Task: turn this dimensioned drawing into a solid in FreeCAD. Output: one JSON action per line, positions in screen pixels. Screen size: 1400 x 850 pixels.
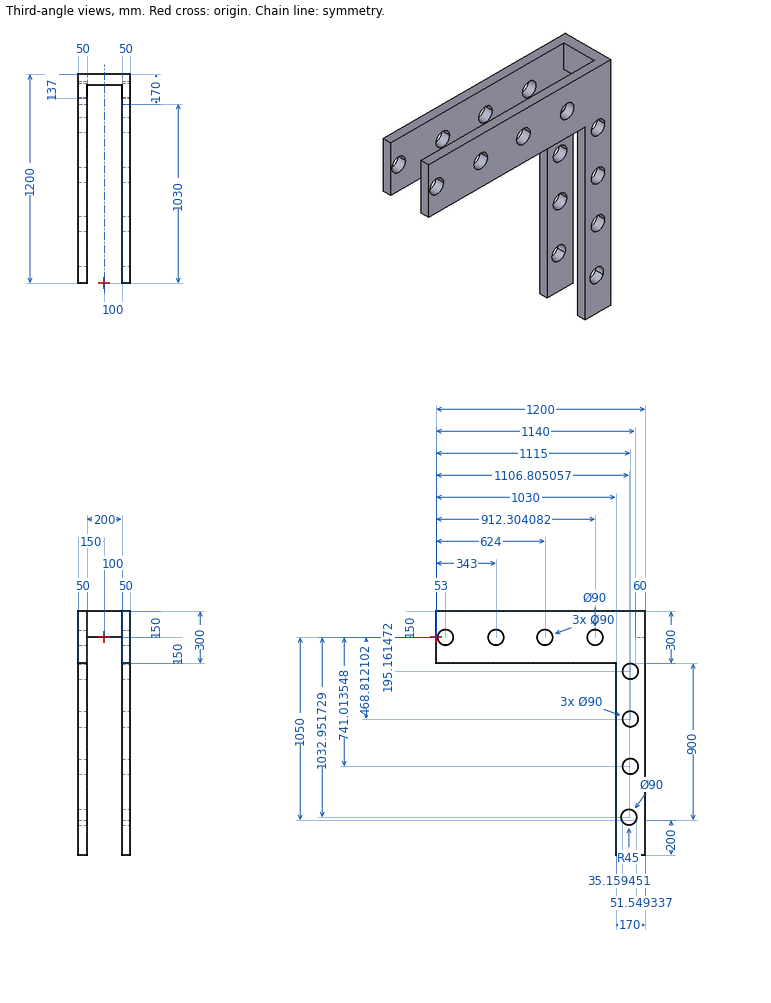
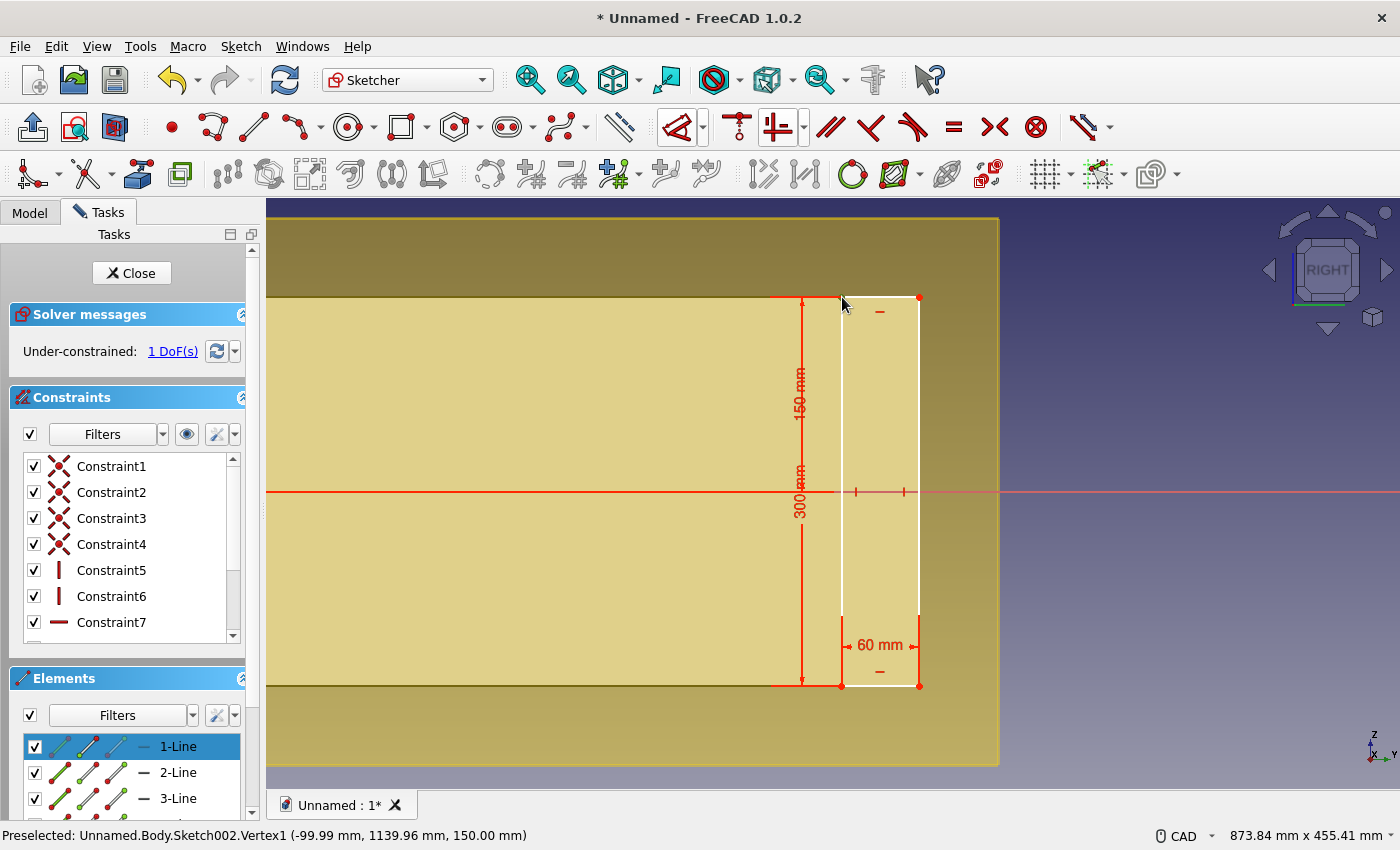
{"action": "left_click", "coordinate": [702, 128]}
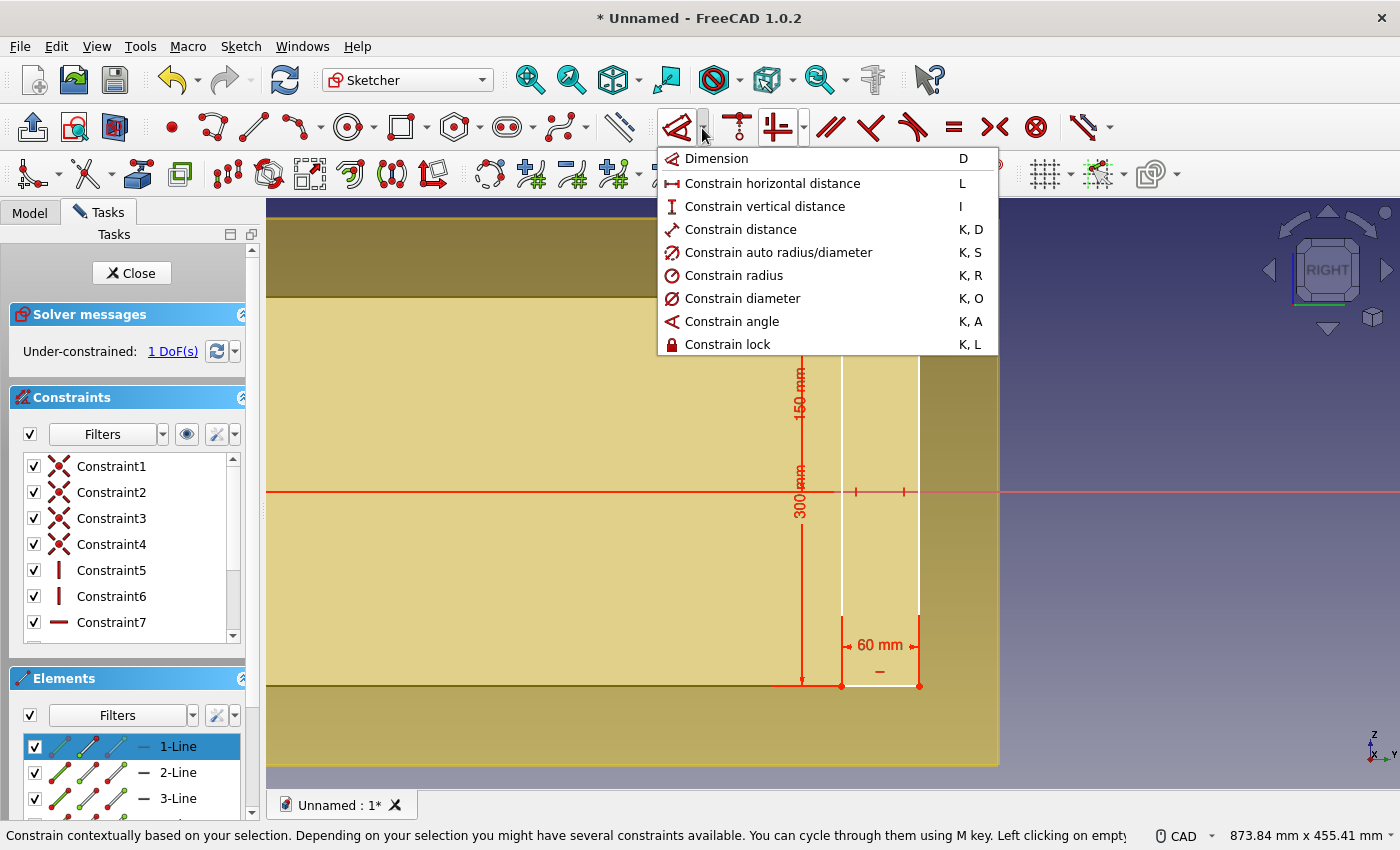
{"action": "left_click", "coordinate": [828, 184]}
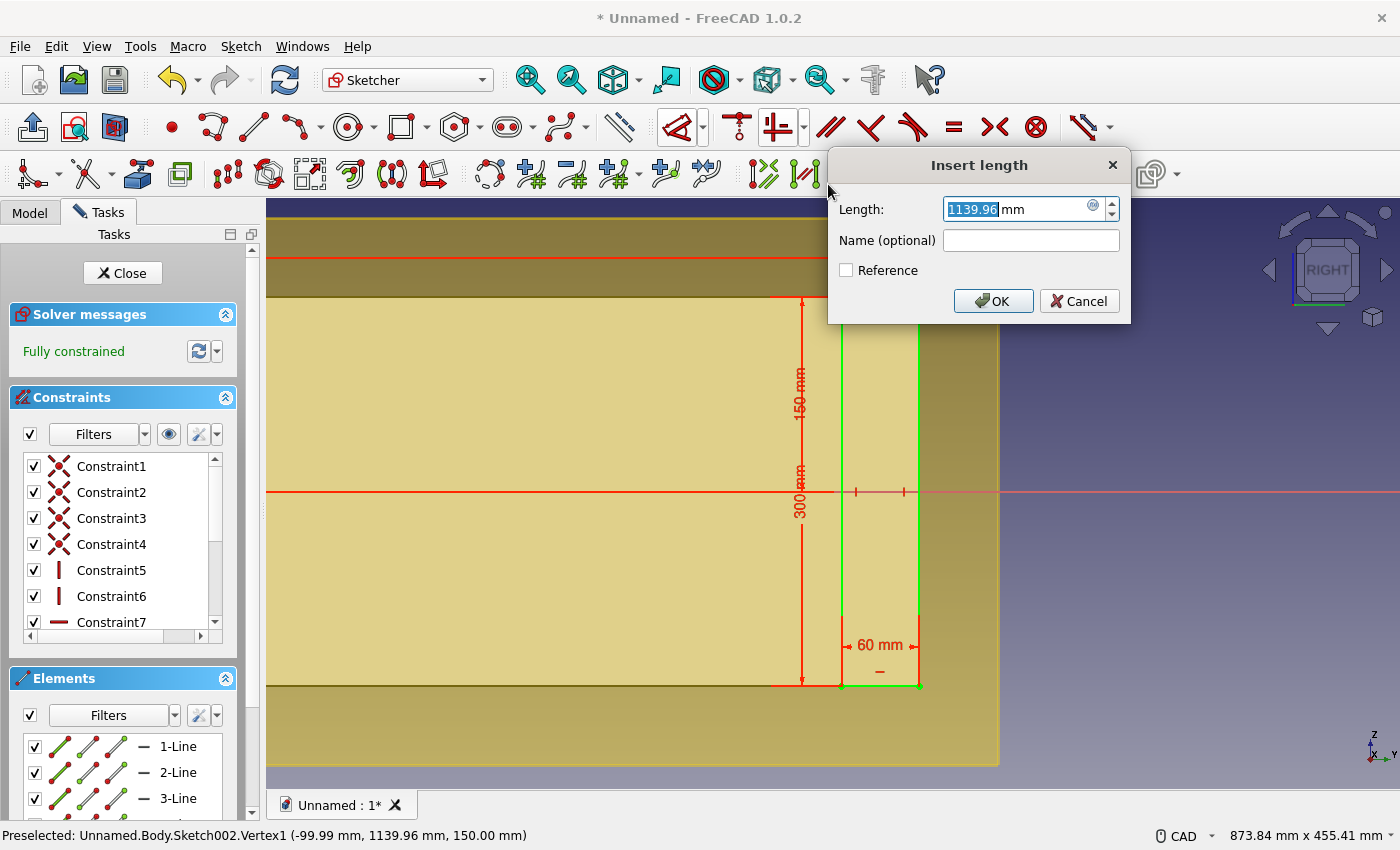
{"action": "type", "text": "1140"}
{"action": "key", "text": "Return"}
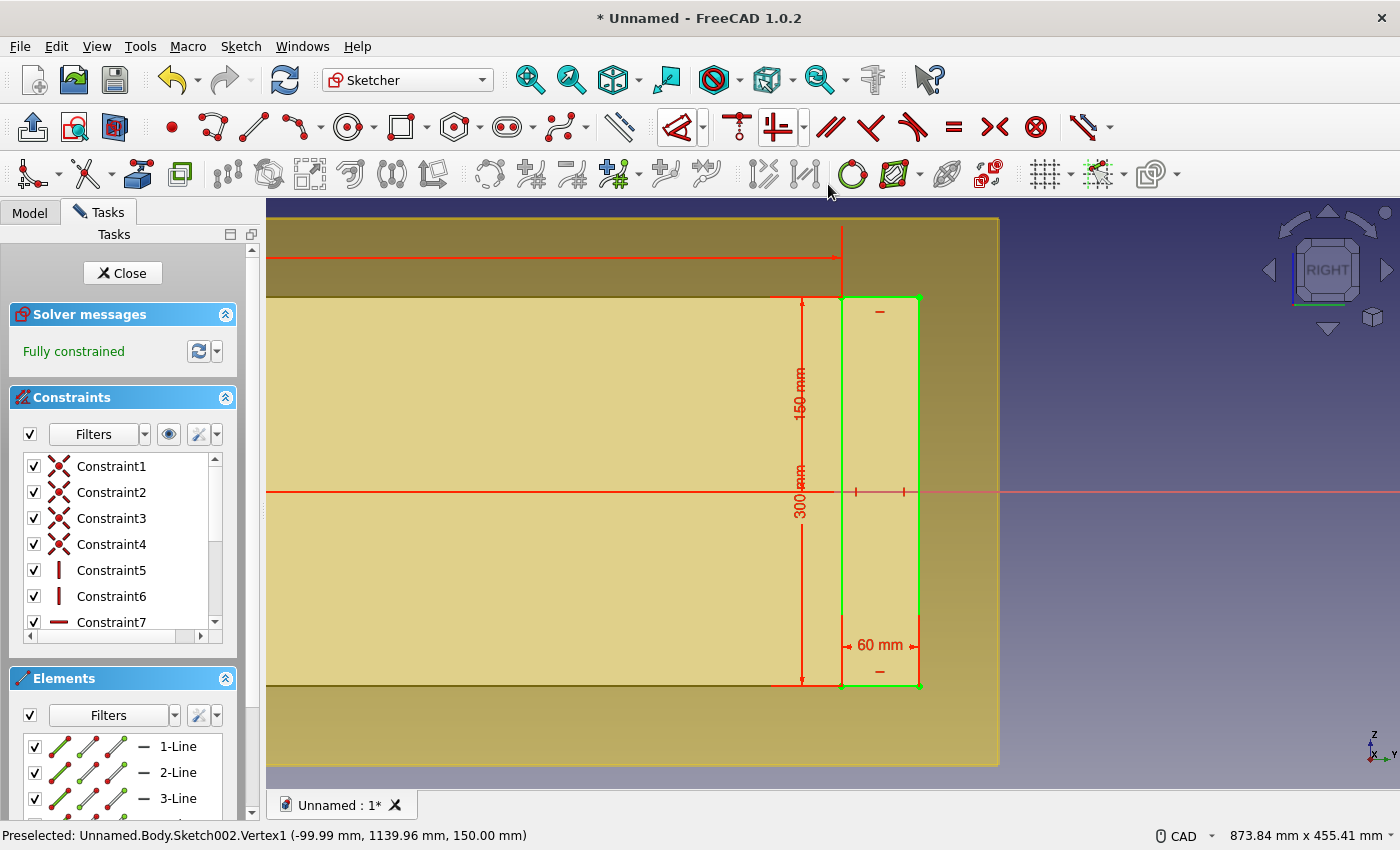
{"action": "left_click", "coordinate": [123, 273]}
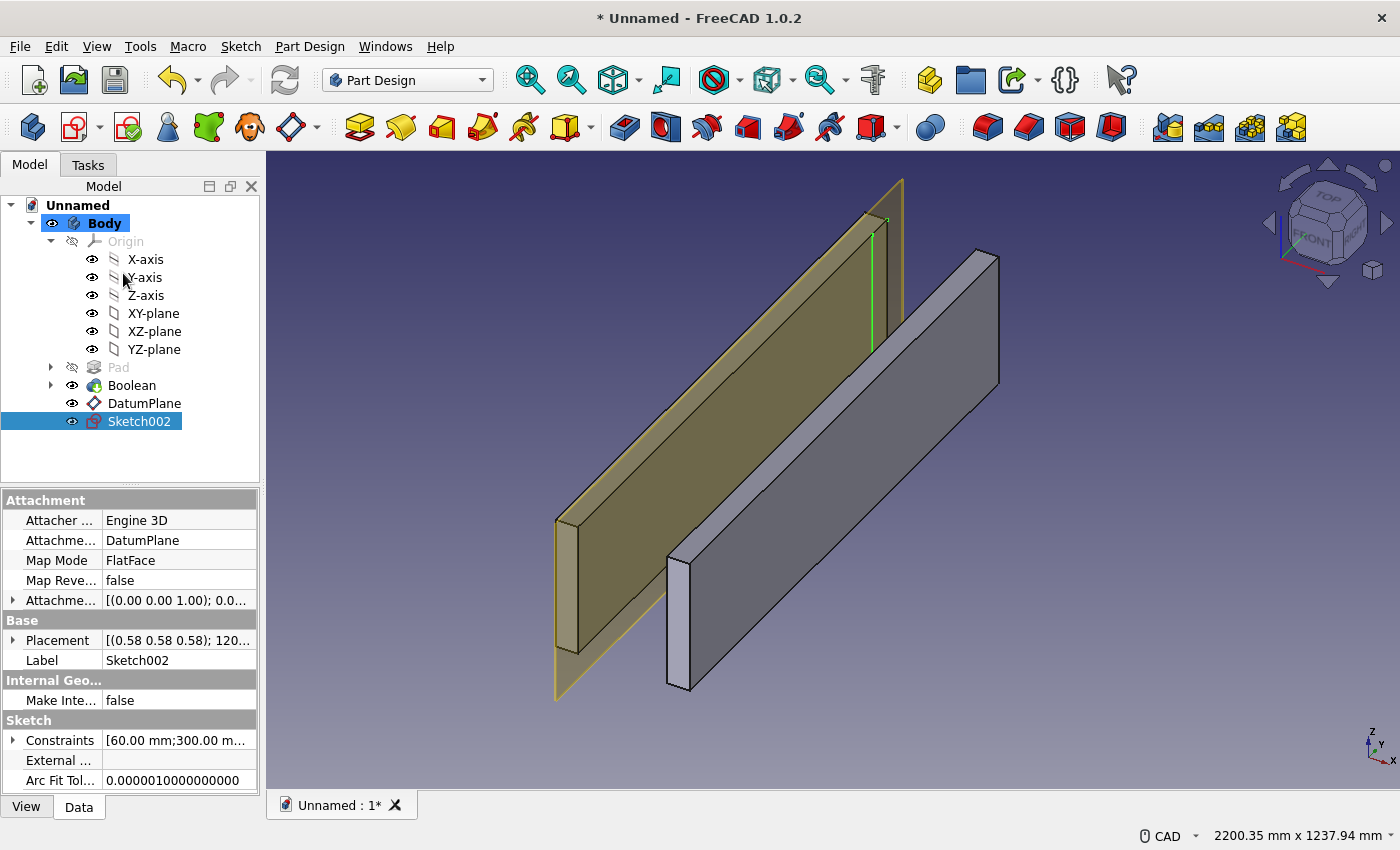
{"action": "left_click", "coordinate": [360, 128]}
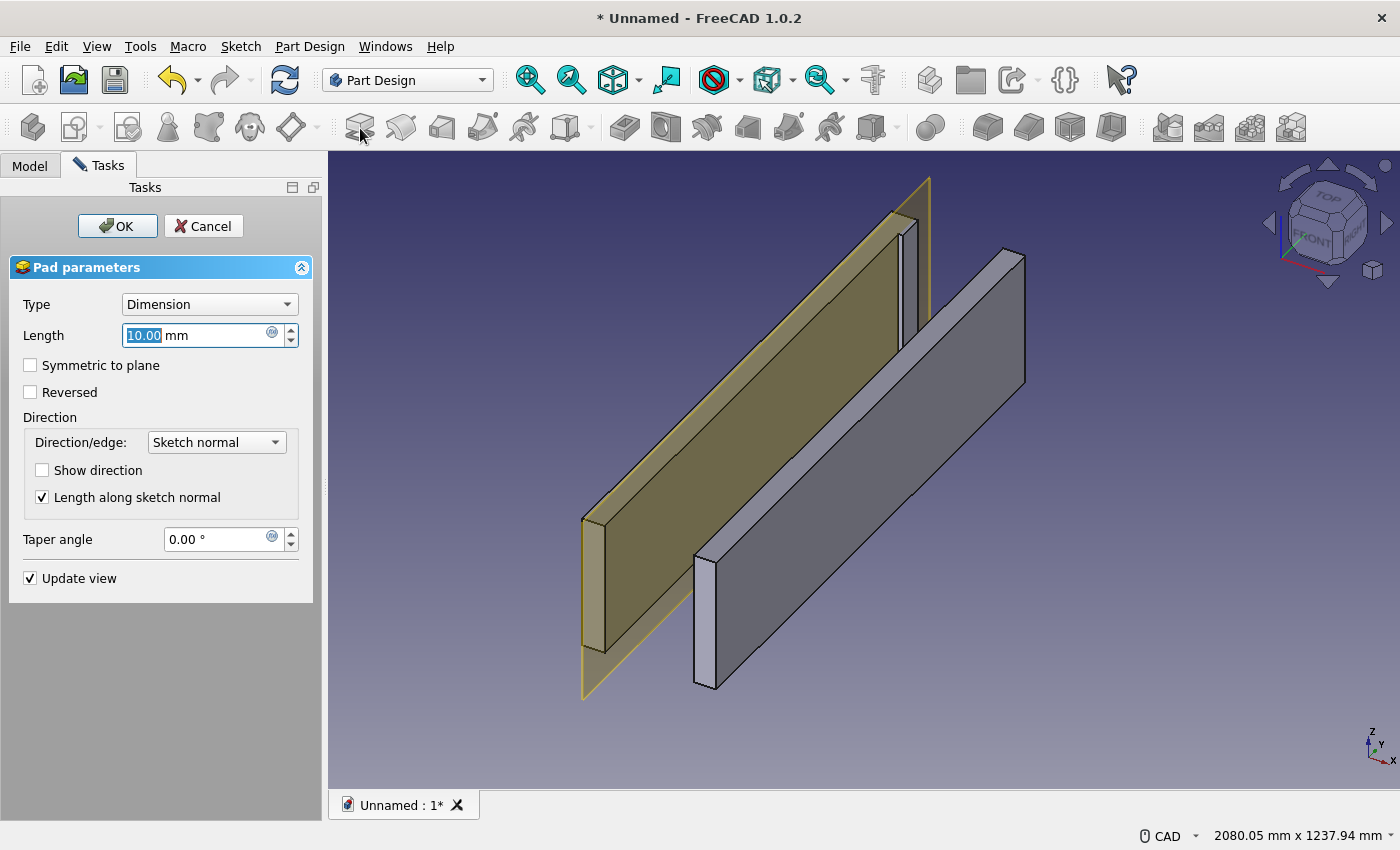
{"action": "left_click", "coordinate": [210, 304]}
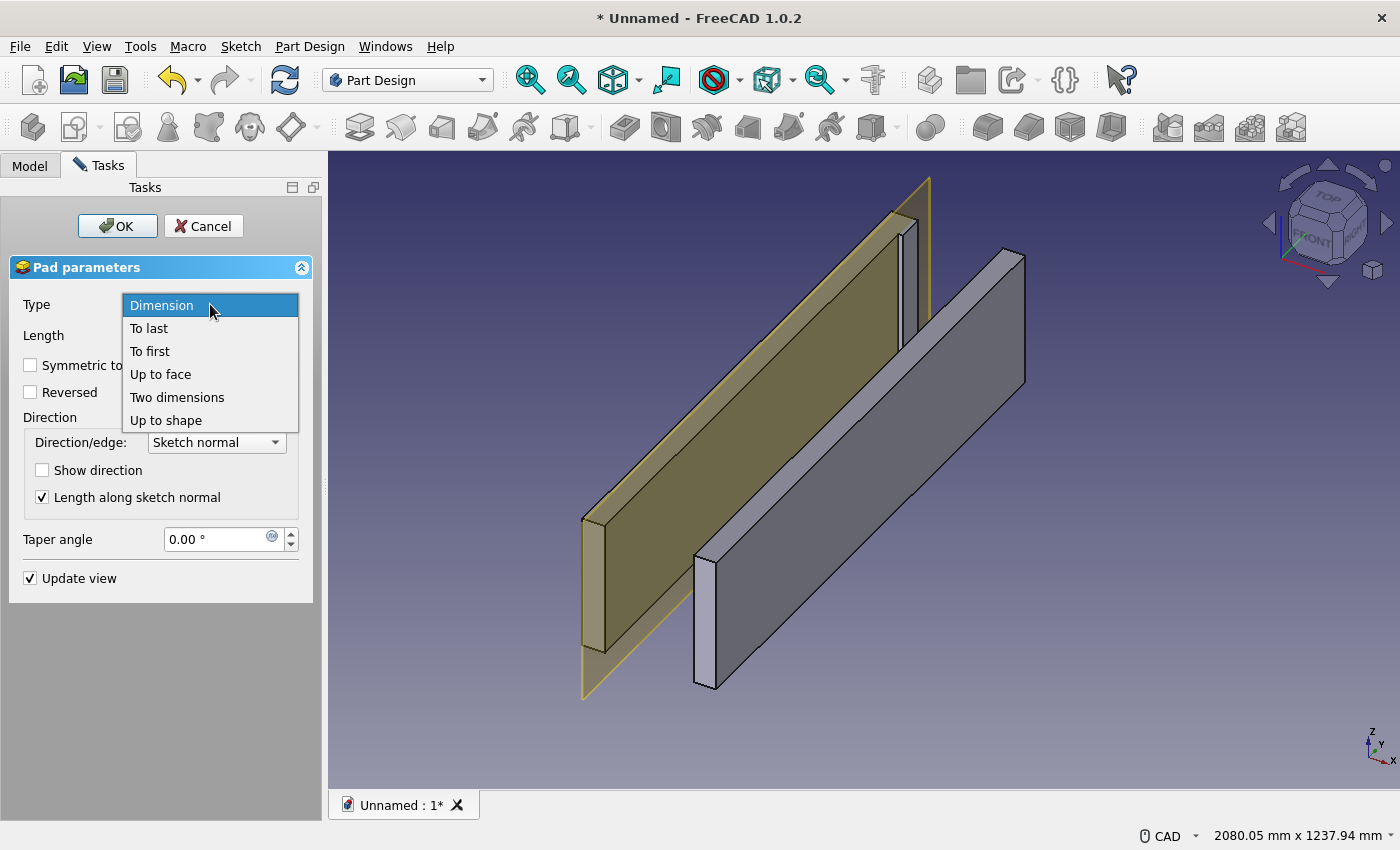
{"action": "left_click", "coordinate": [208, 352]}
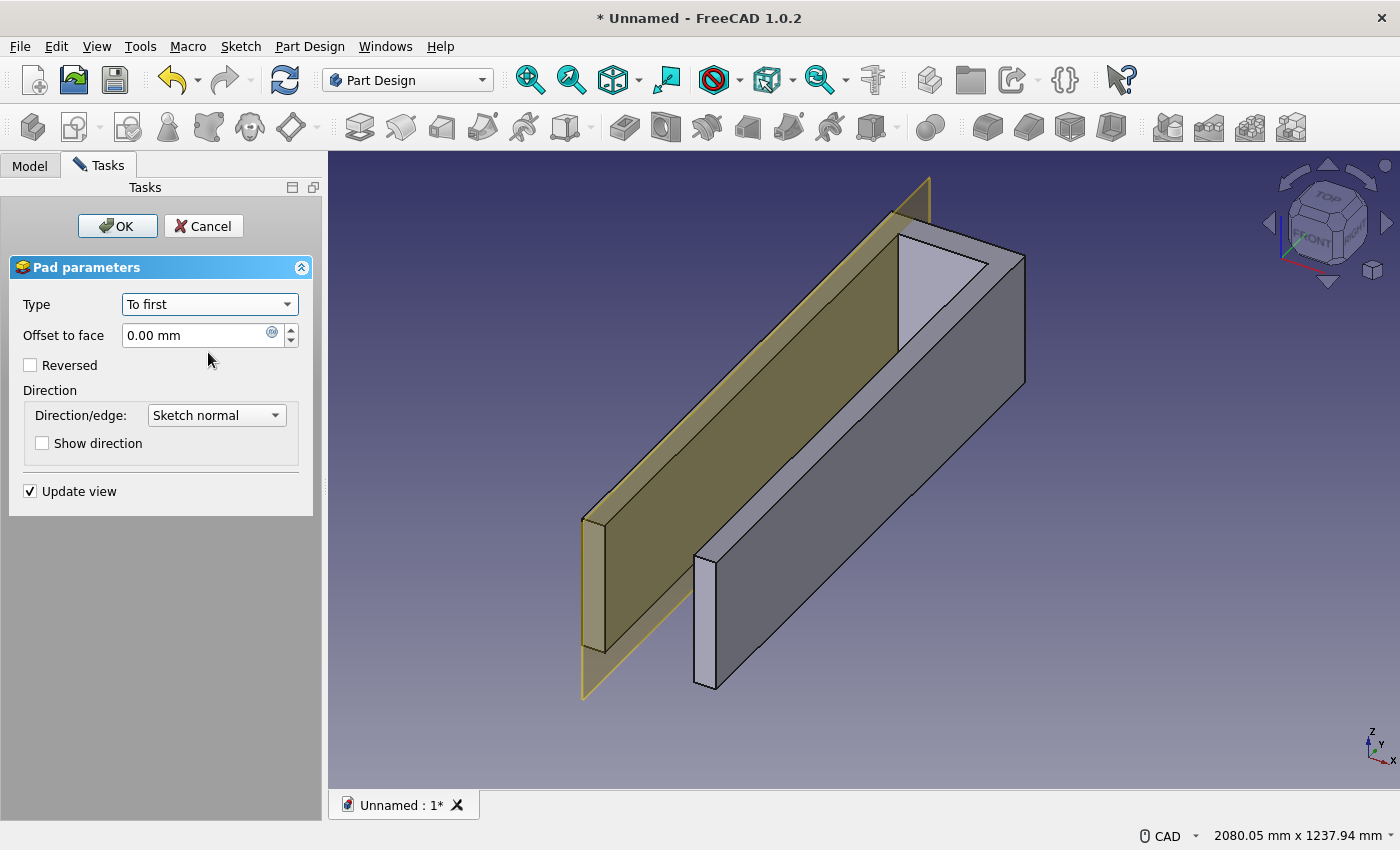
{"action": "left_click", "coordinate": [118, 226]}